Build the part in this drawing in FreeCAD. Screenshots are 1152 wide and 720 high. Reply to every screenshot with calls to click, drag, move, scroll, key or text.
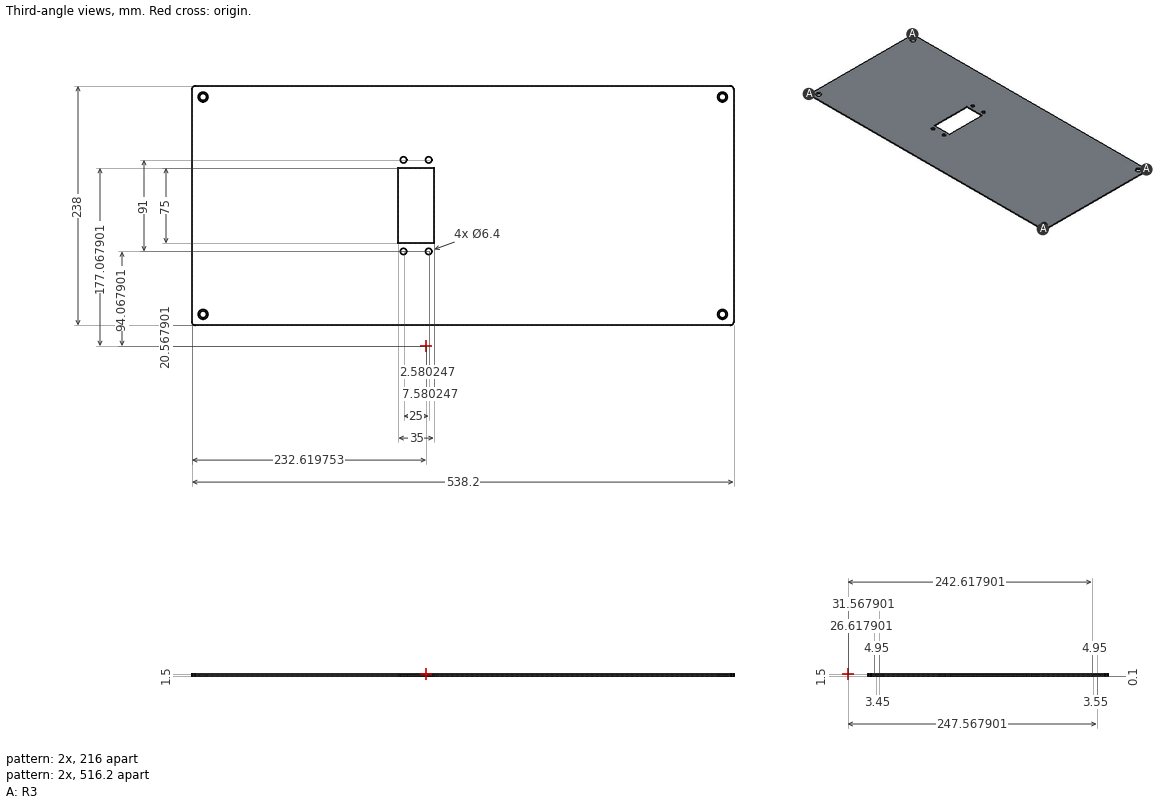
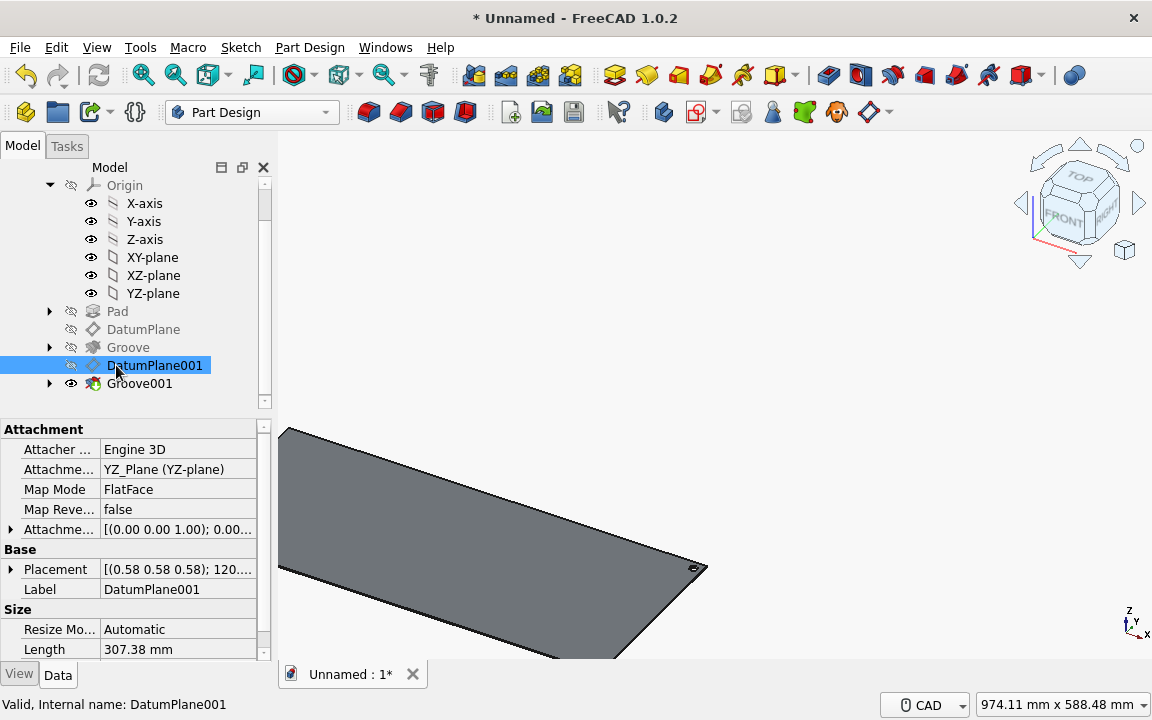
click(144, 76)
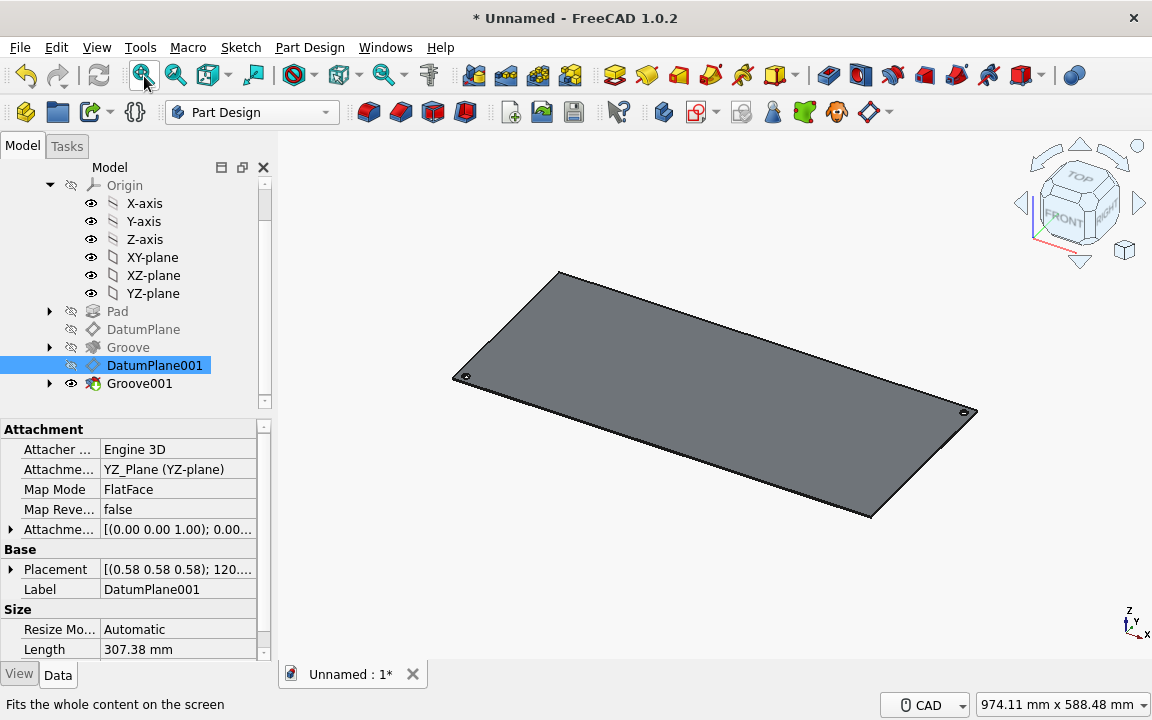
click(116, 383)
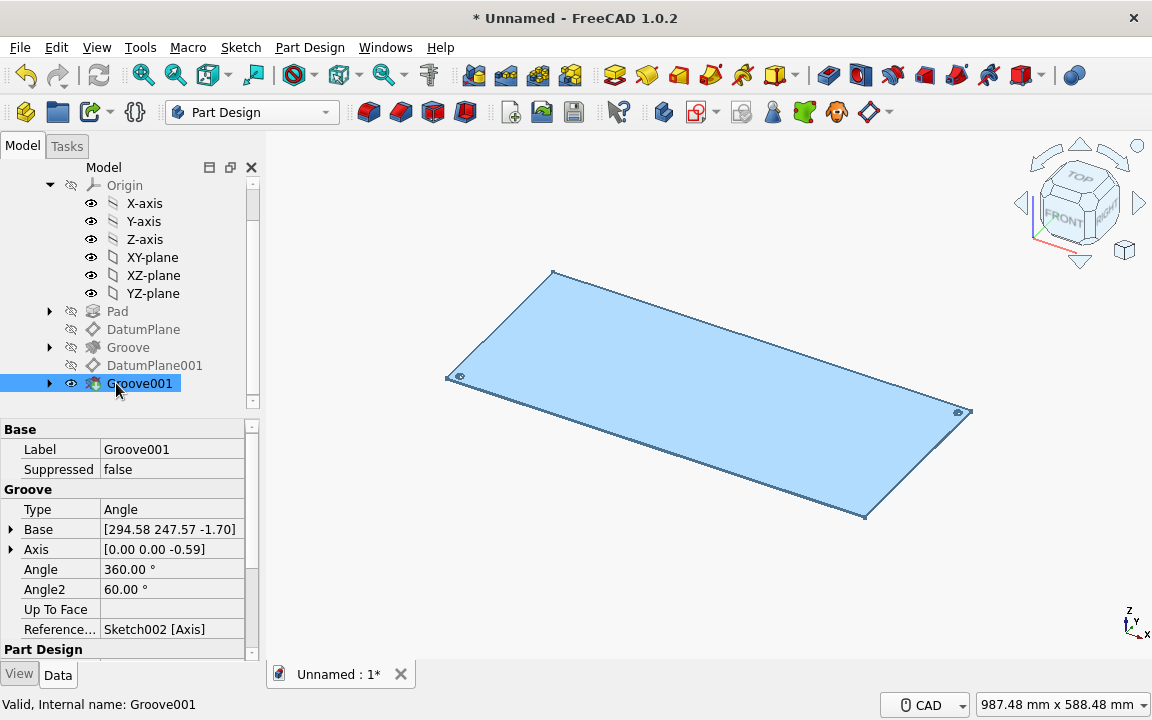
click(506, 76)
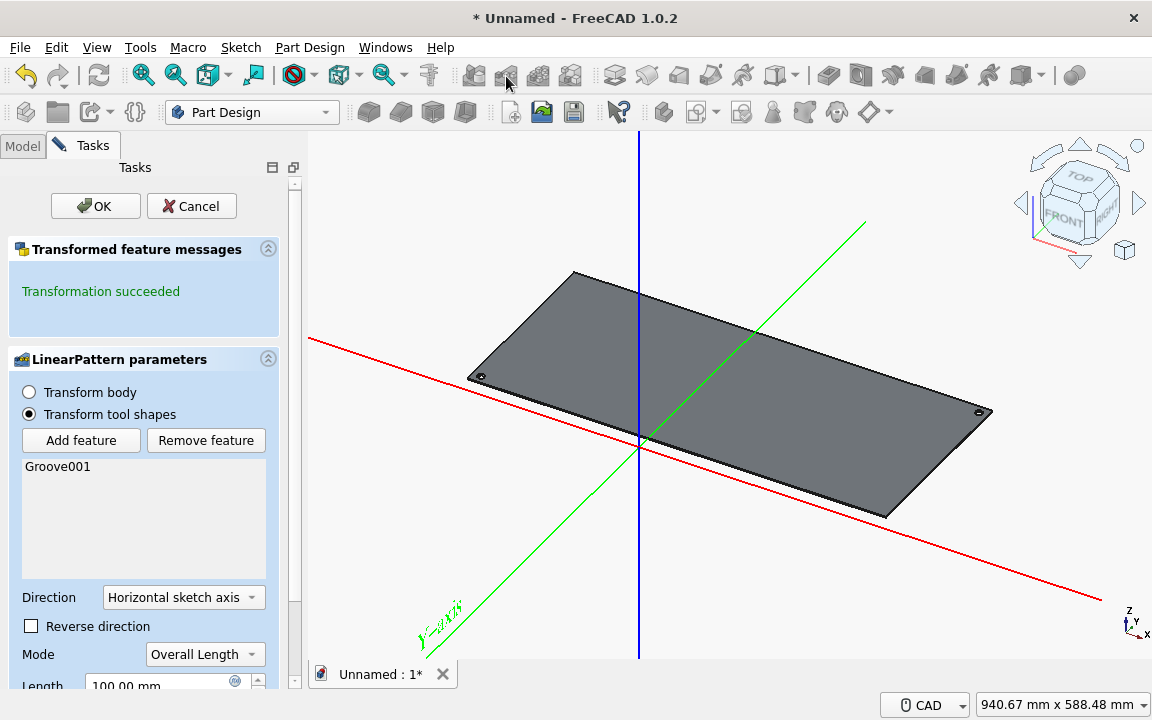
click(184, 598)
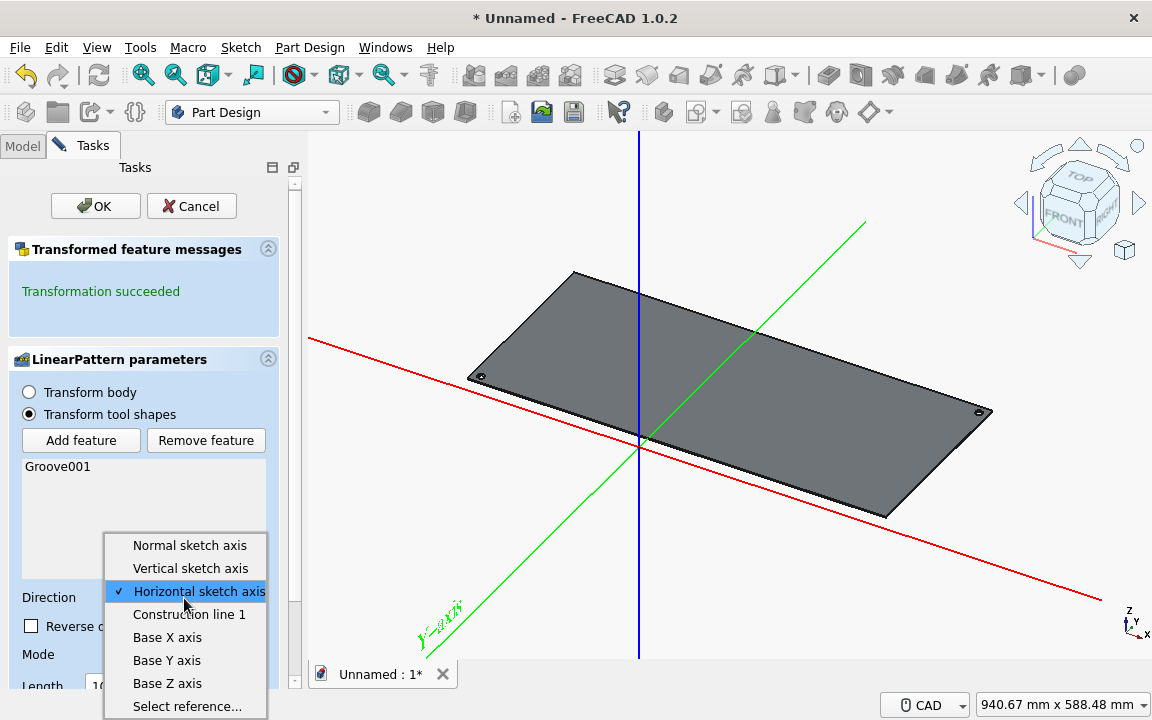
click(184, 660)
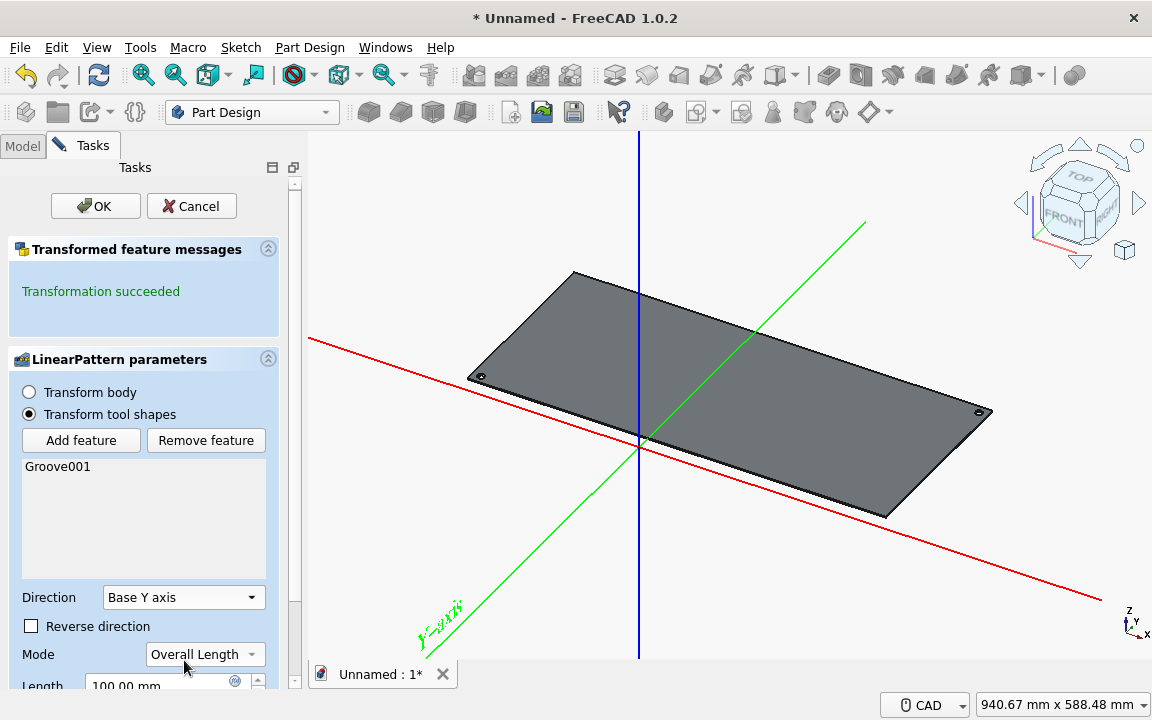
click(206, 654)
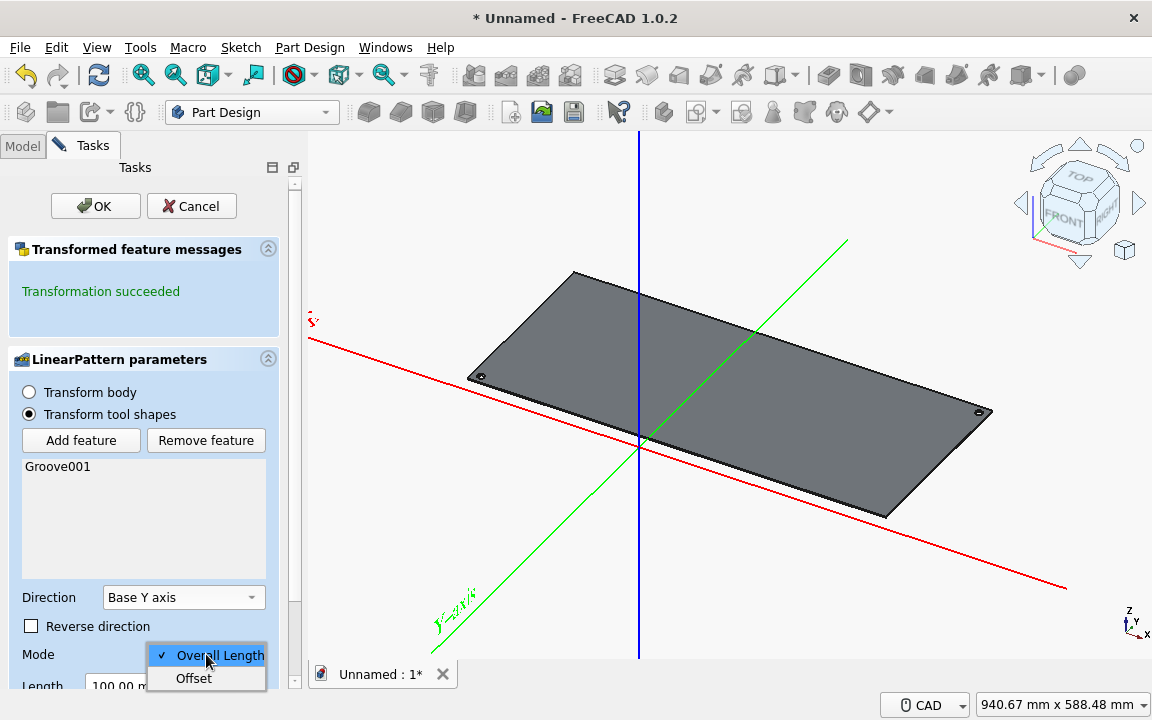
click(206, 678)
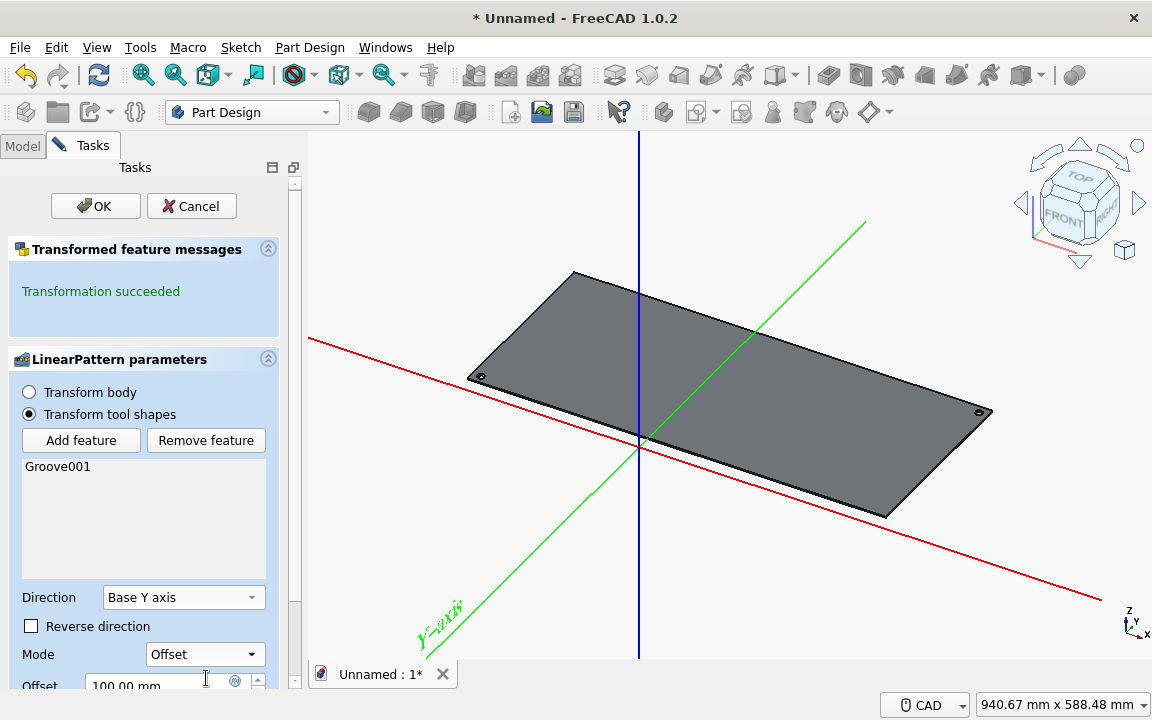
scroll(295, 432, down, 2)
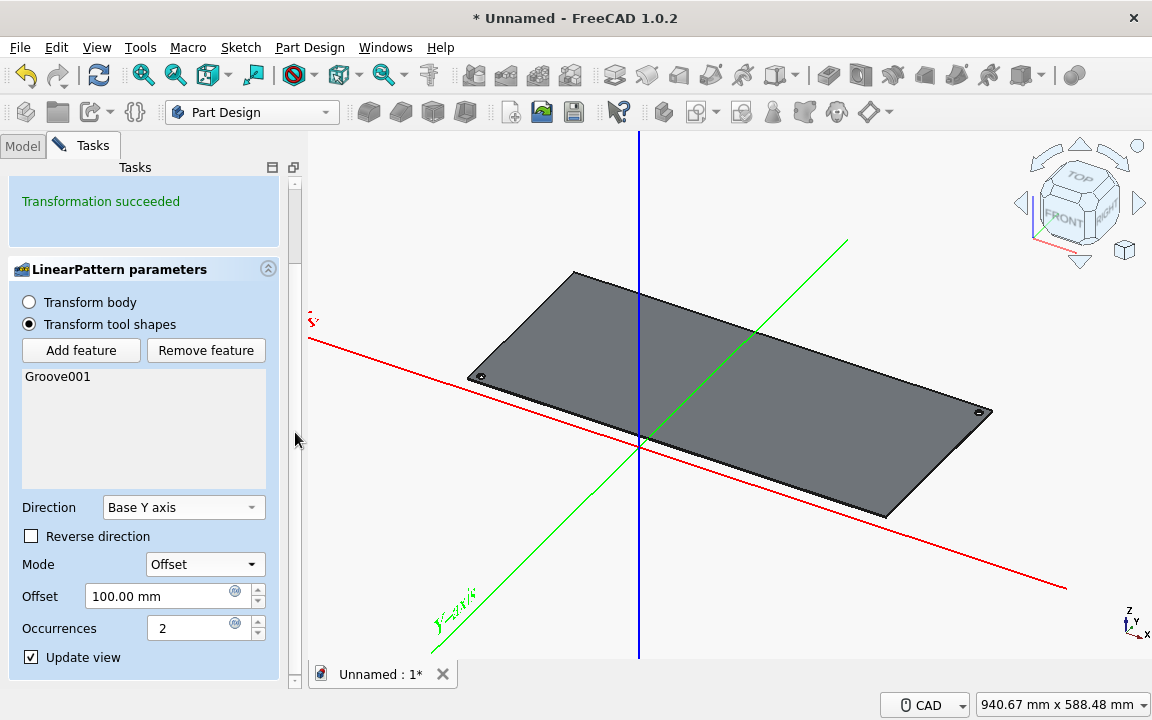
triple_click(168, 596)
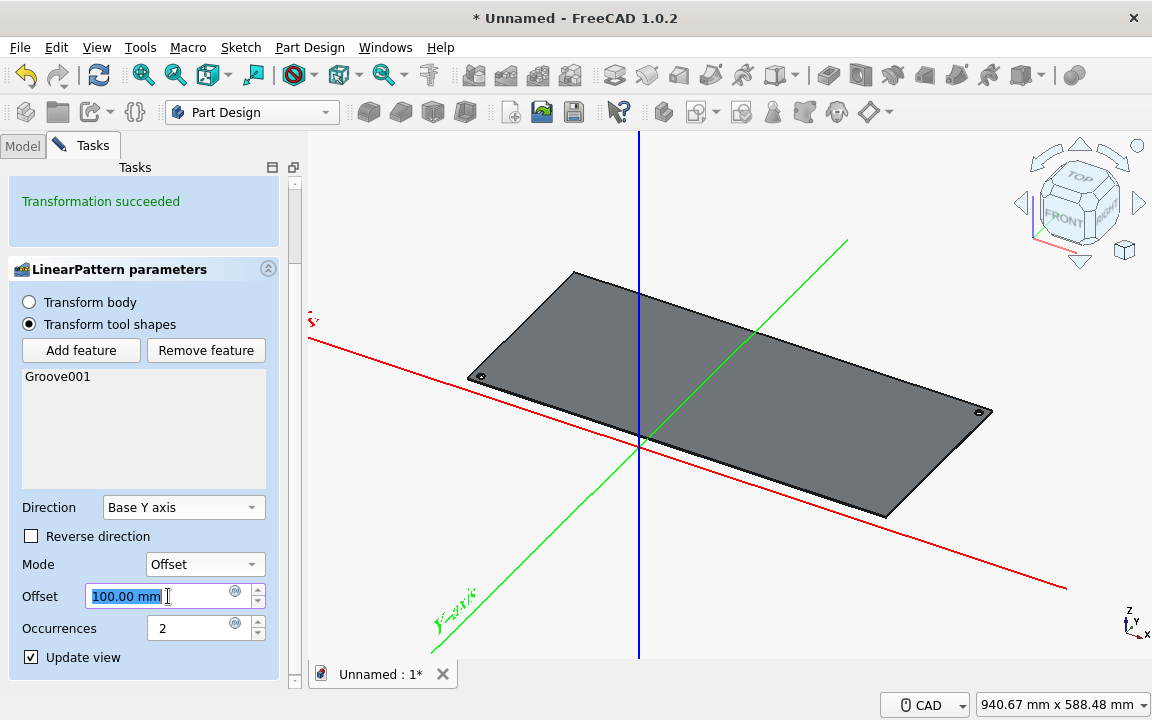
text(216)
key(Tab)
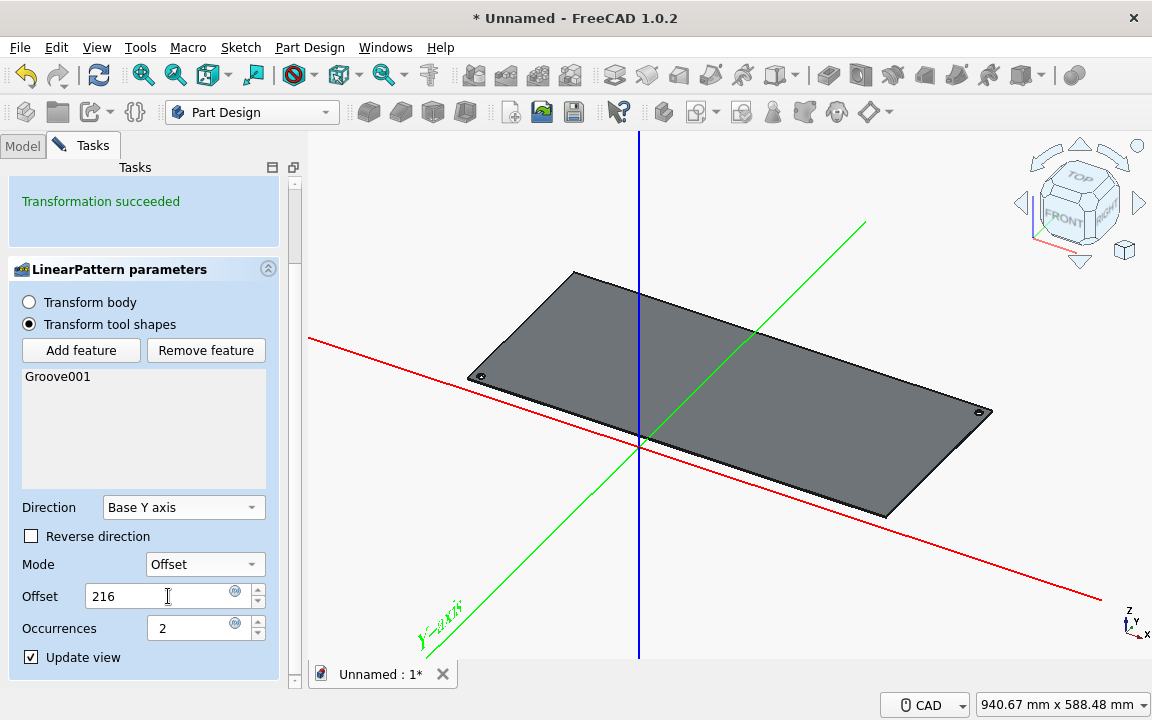
triple_click(198, 628)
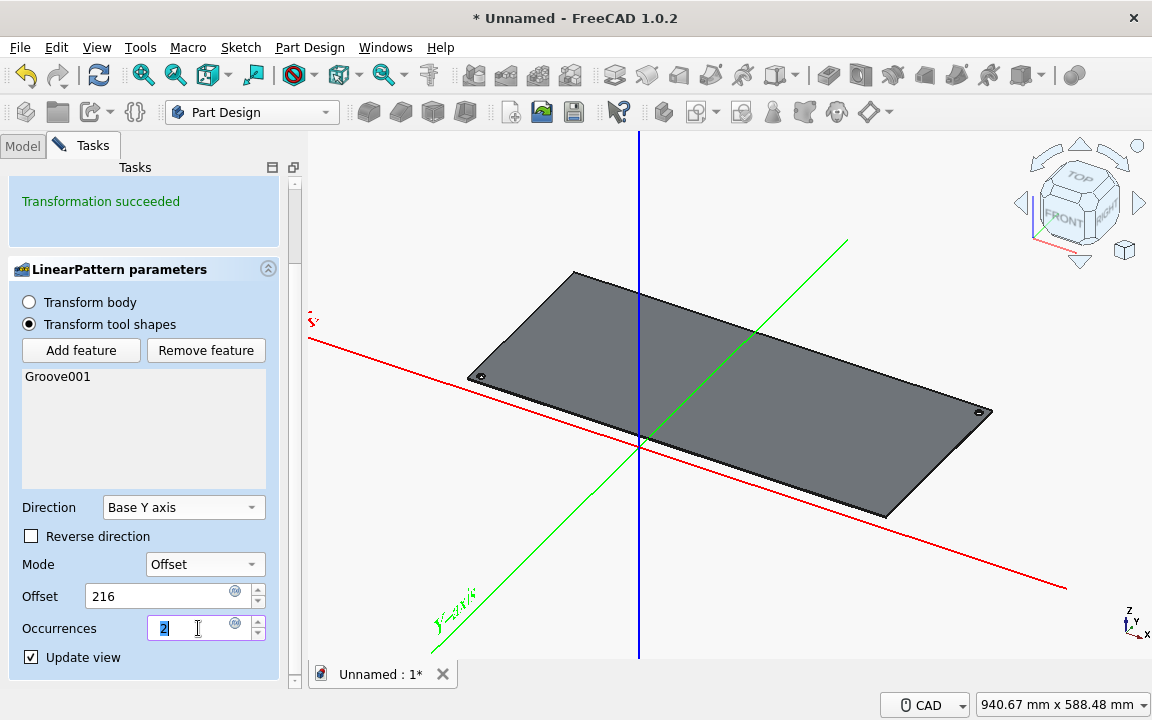
text(2)
key(Tab)